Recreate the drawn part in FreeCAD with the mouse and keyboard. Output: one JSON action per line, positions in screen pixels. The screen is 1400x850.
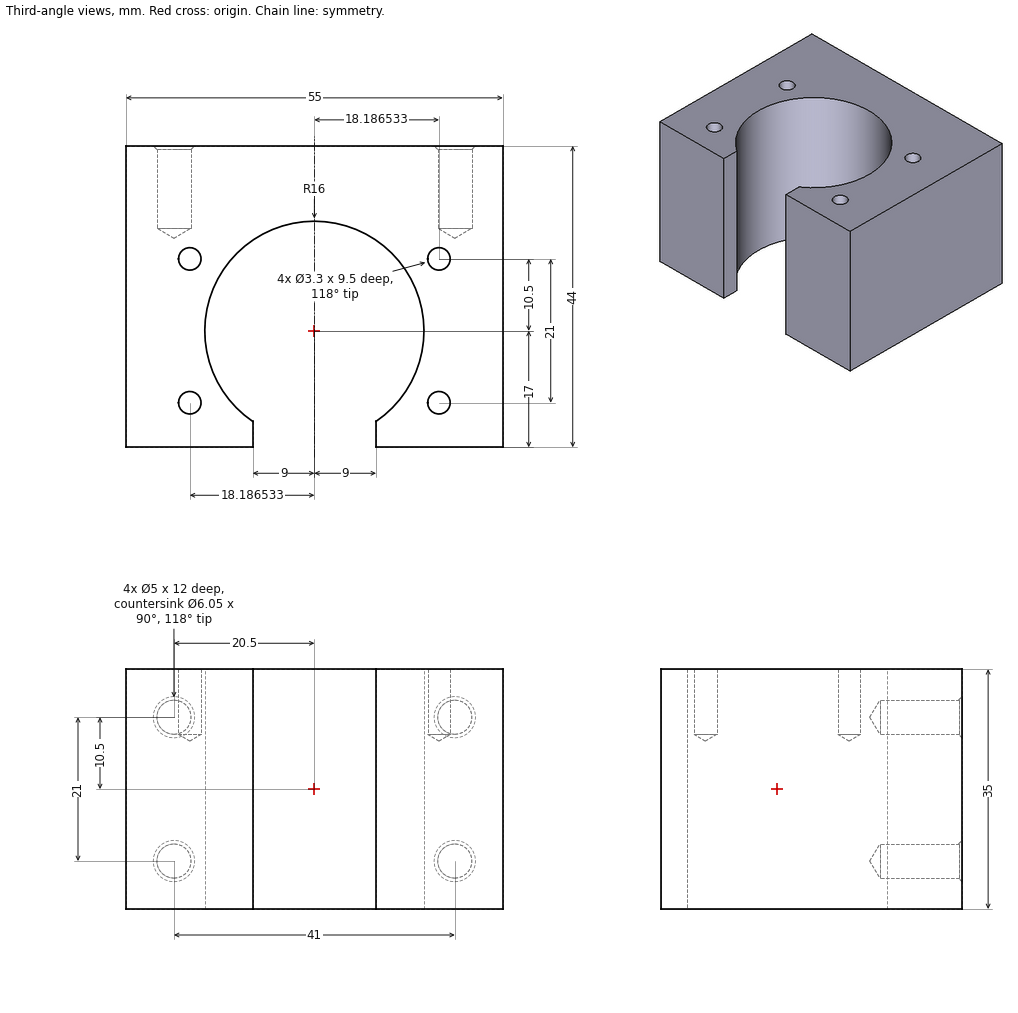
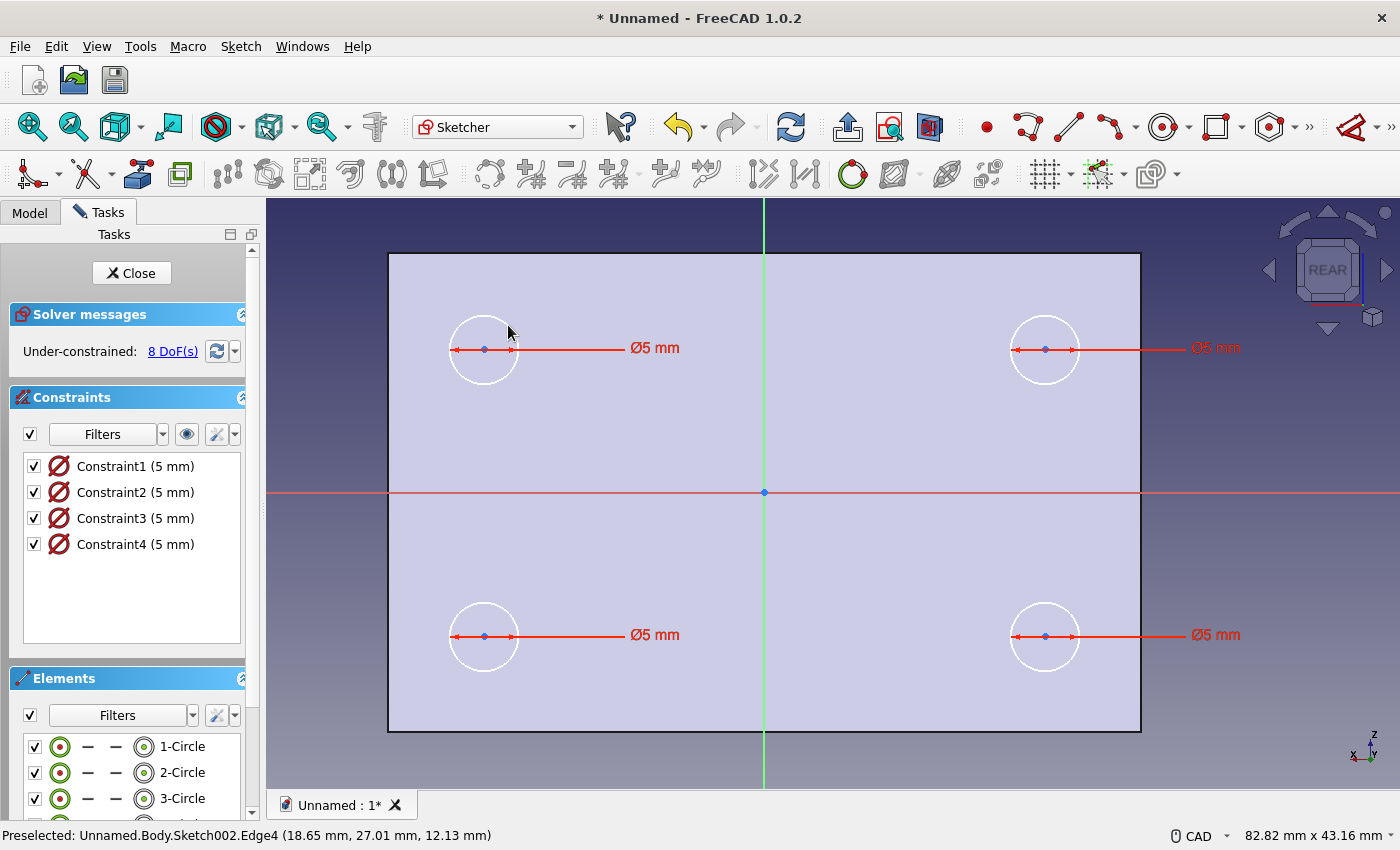
{"action": "left_click", "coordinate": [1045, 350]}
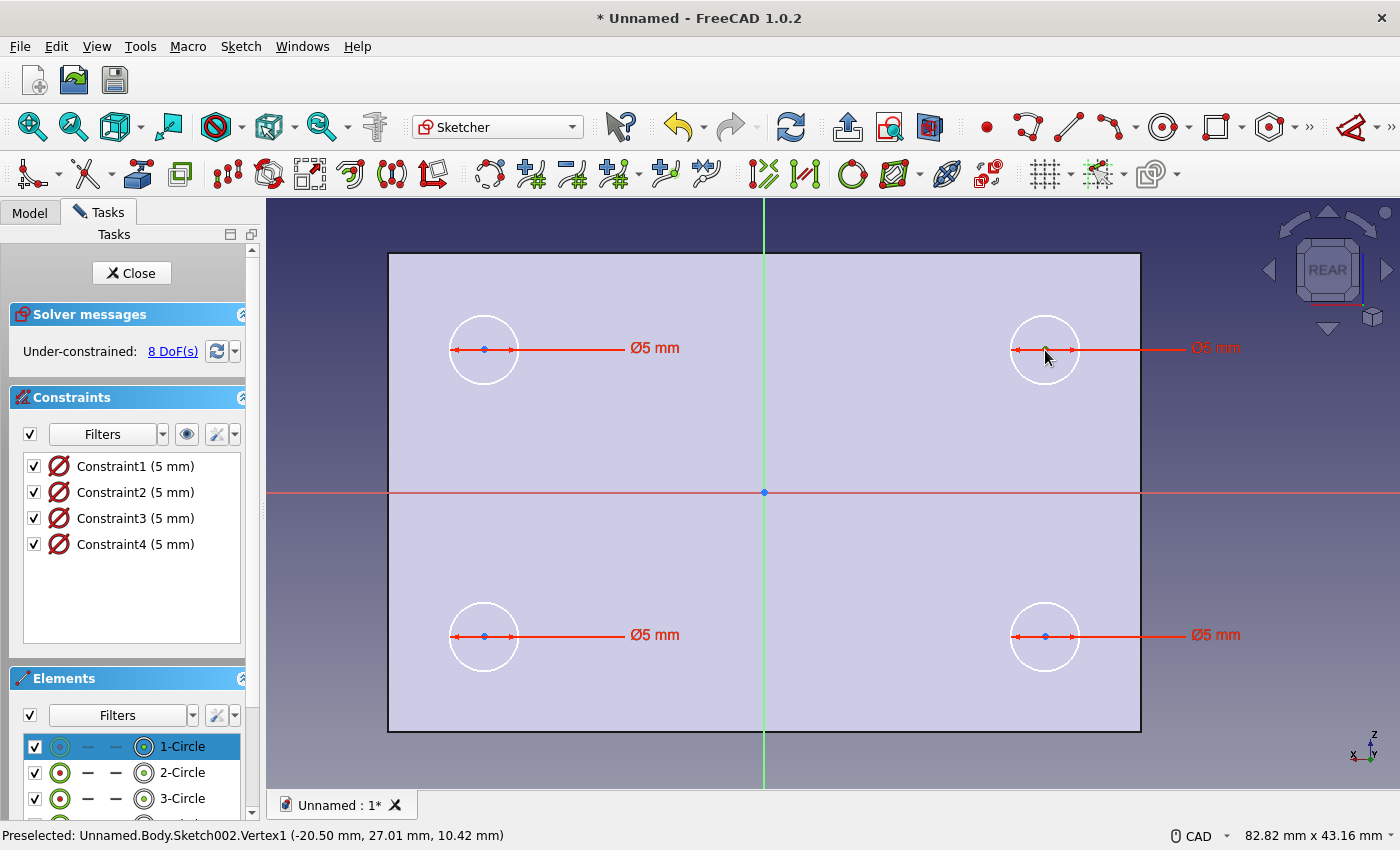
{"action": "left_click", "coordinate": [1045, 637]}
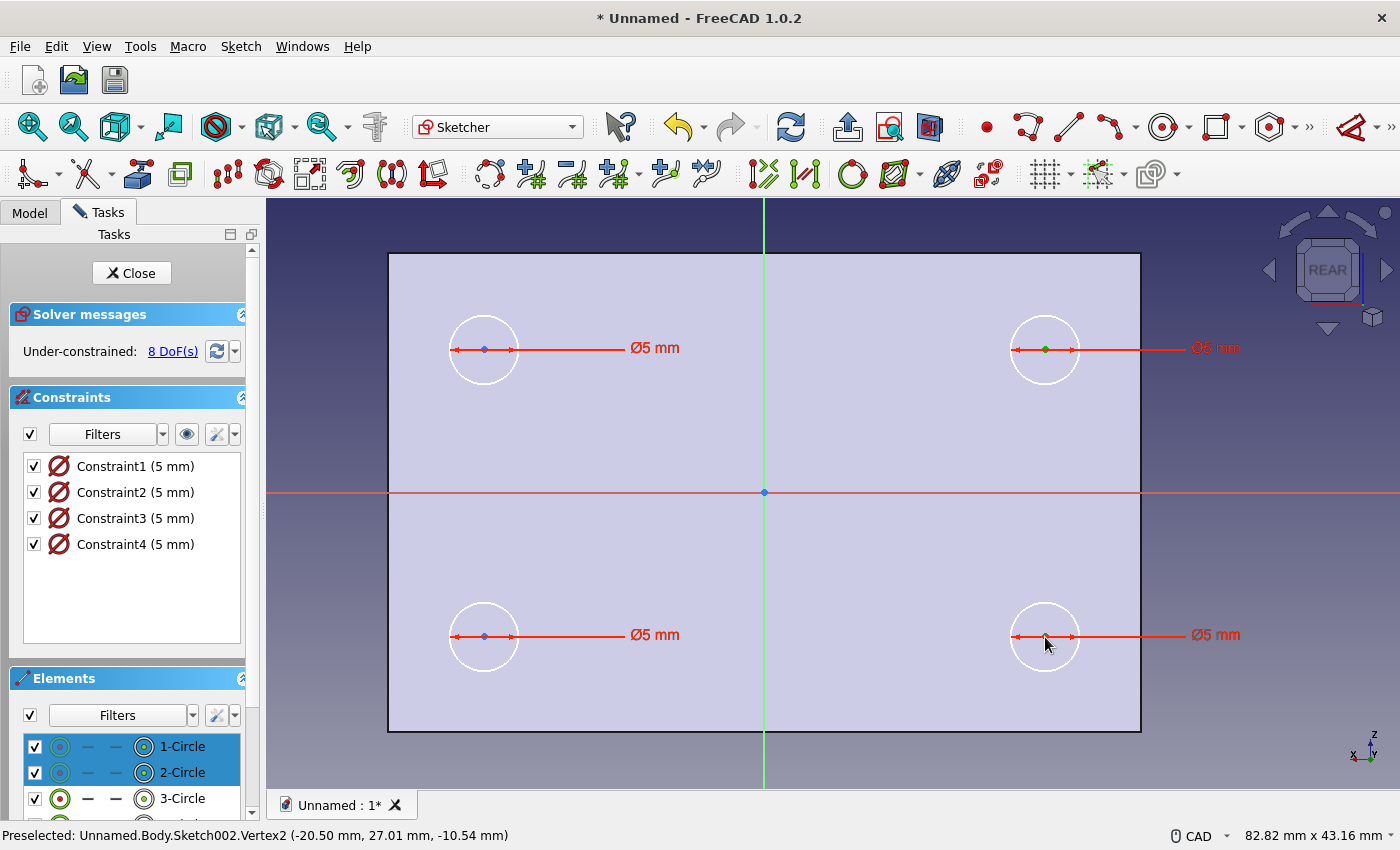
{"action": "key", "text": "v"}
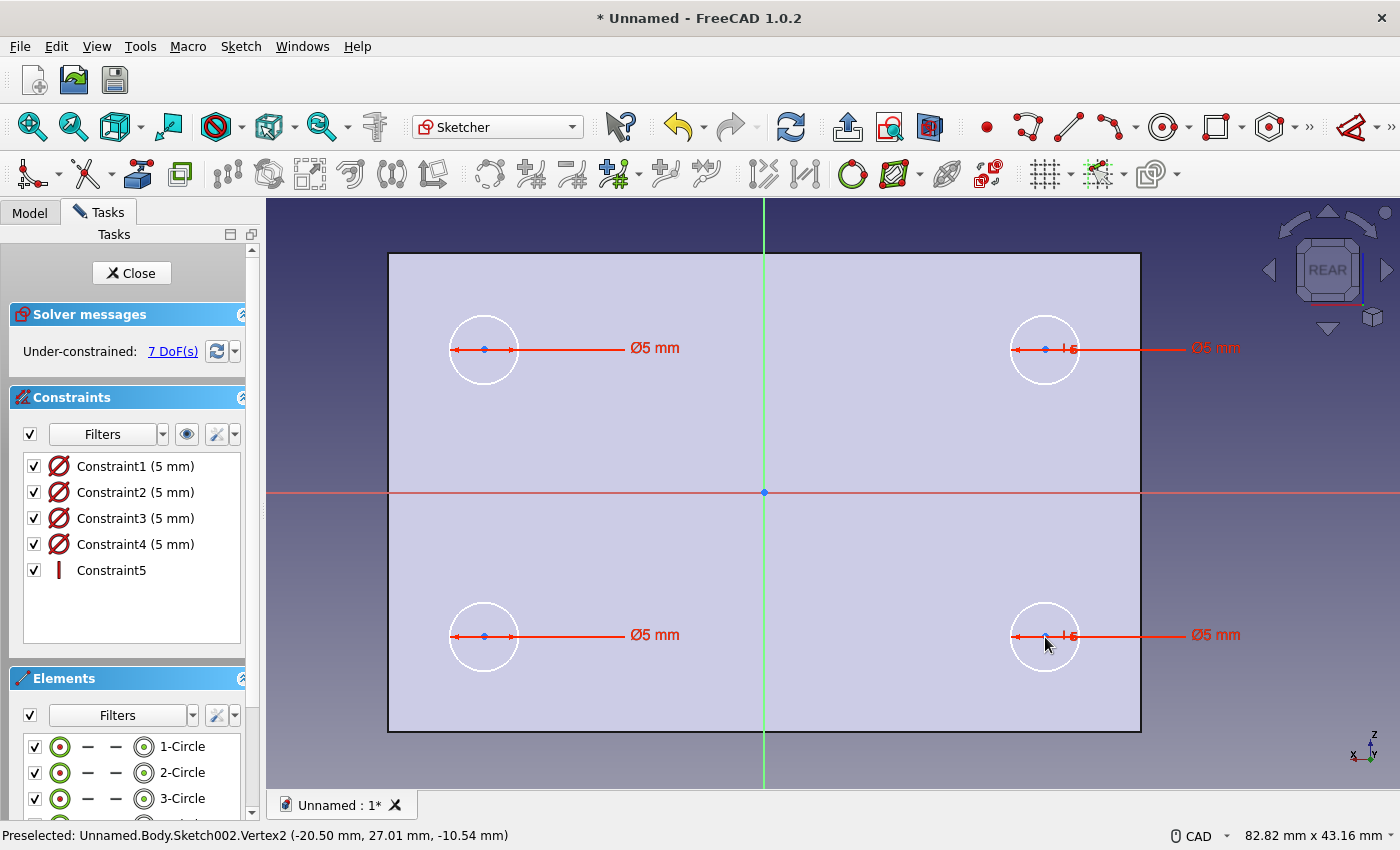
{"action": "left_click", "coordinate": [1045, 637]}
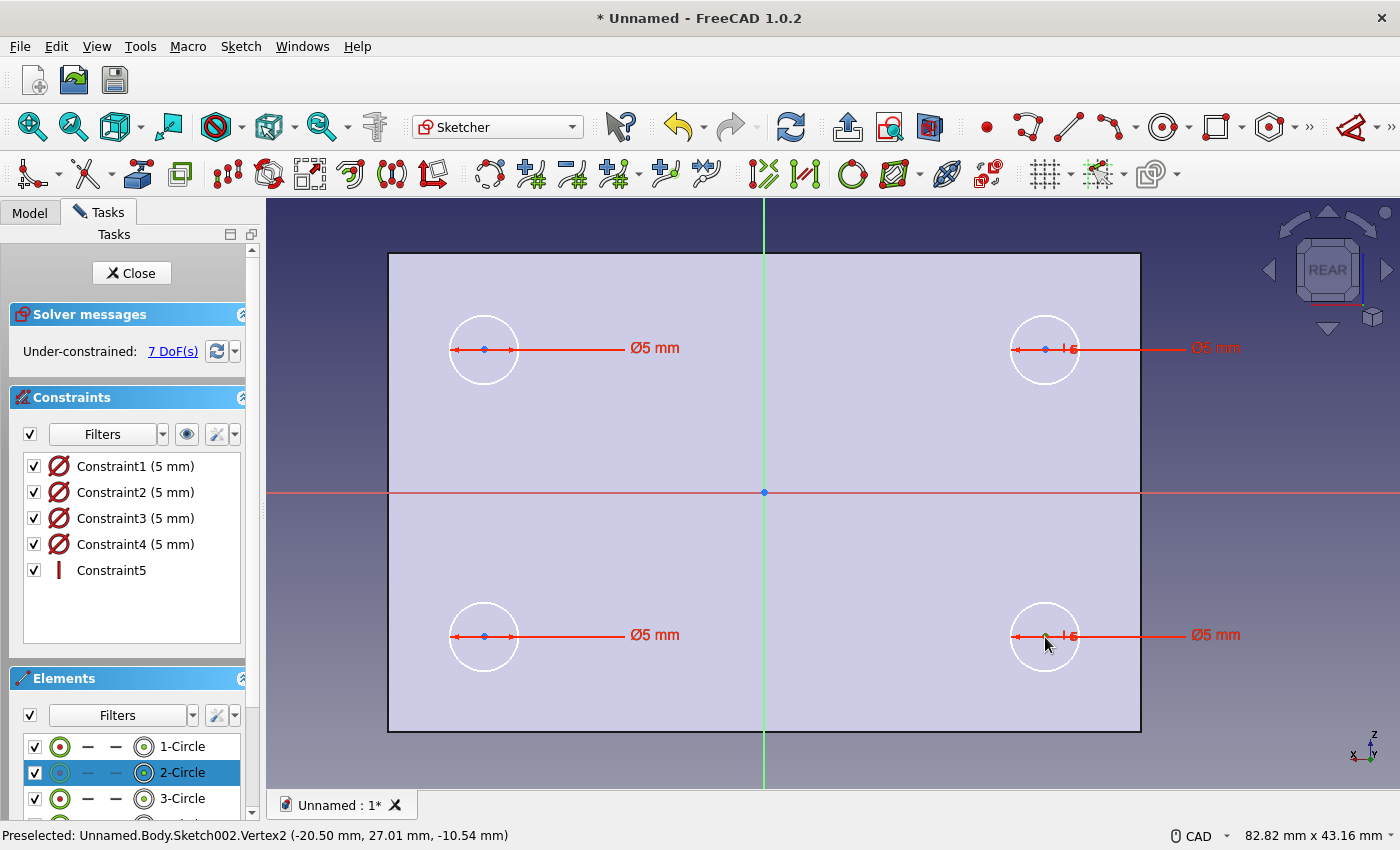
{"action": "left_click", "coordinate": [484, 637]}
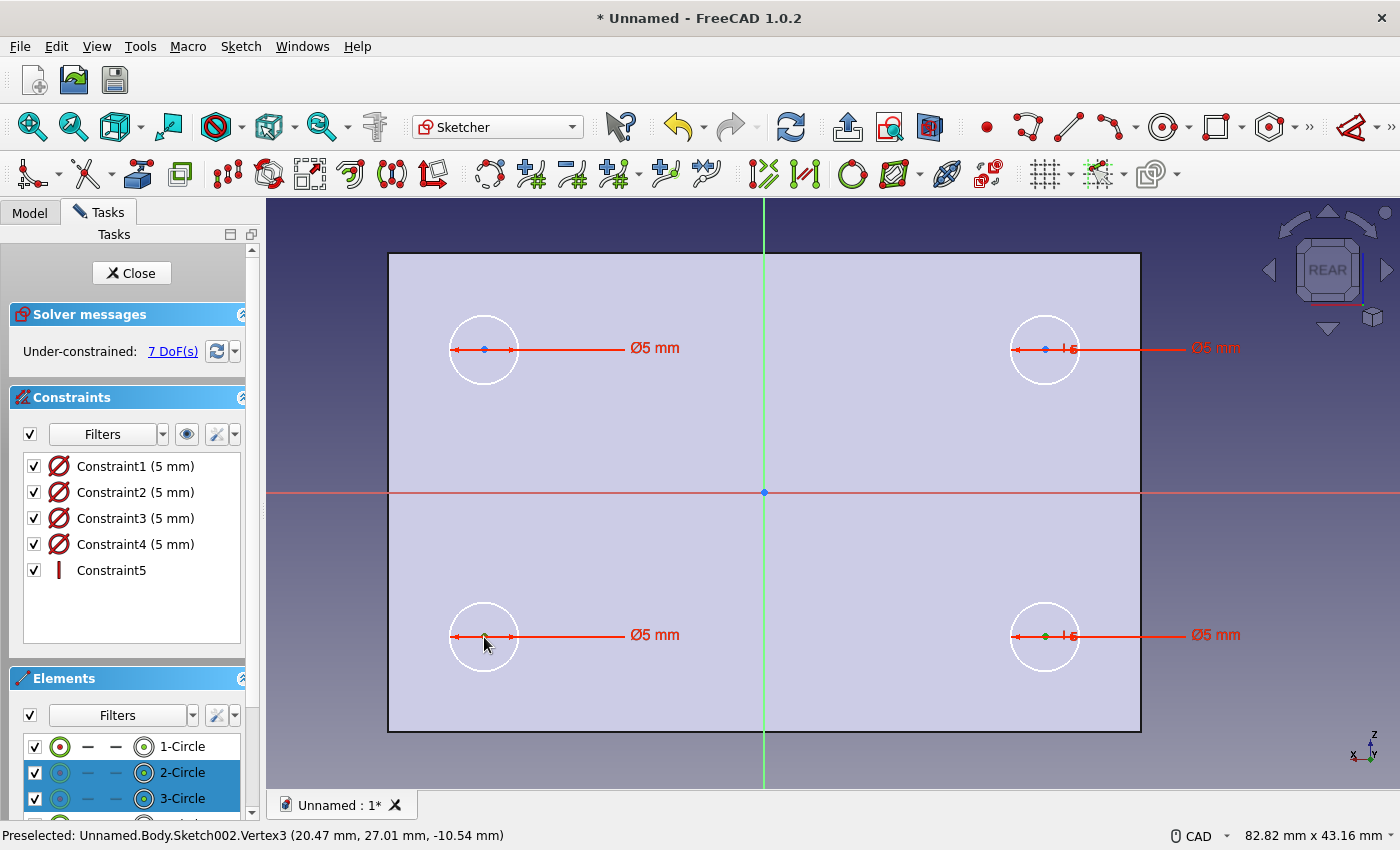
{"action": "key", "text": "h"}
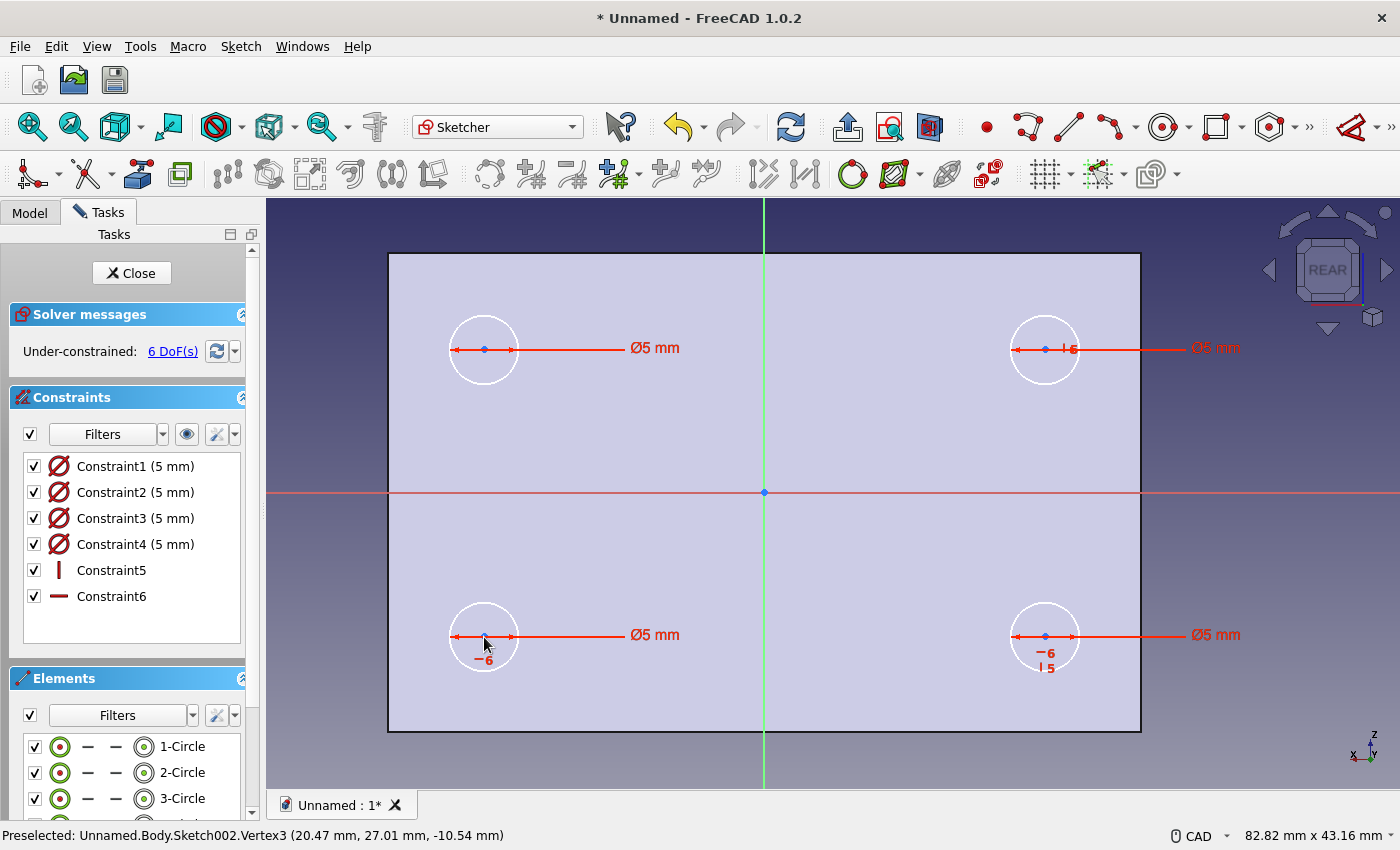
{"action": "left_click", "coordinate": [484, 637]}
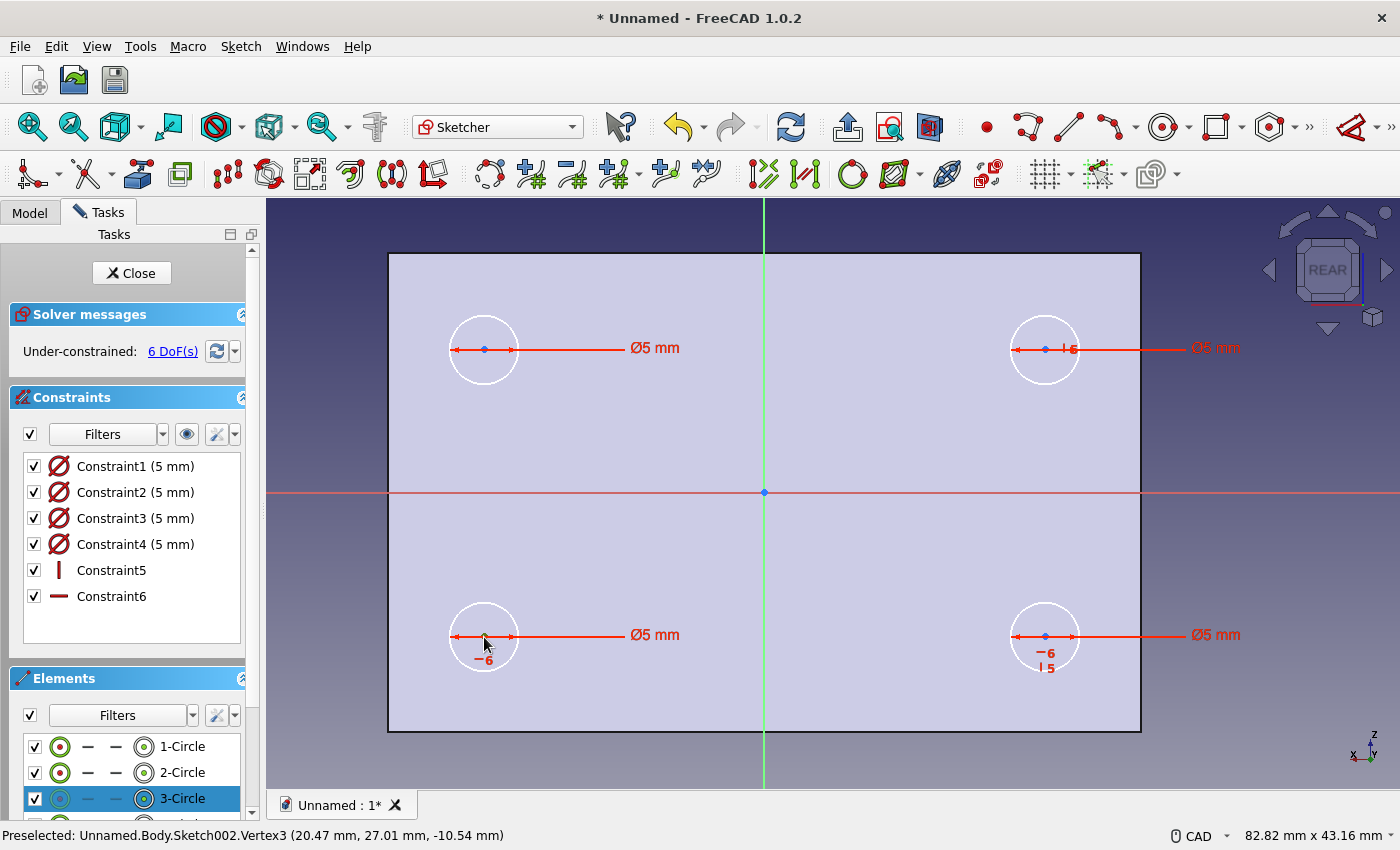
{"action": "left_click", "coordinate": [484, 350]}